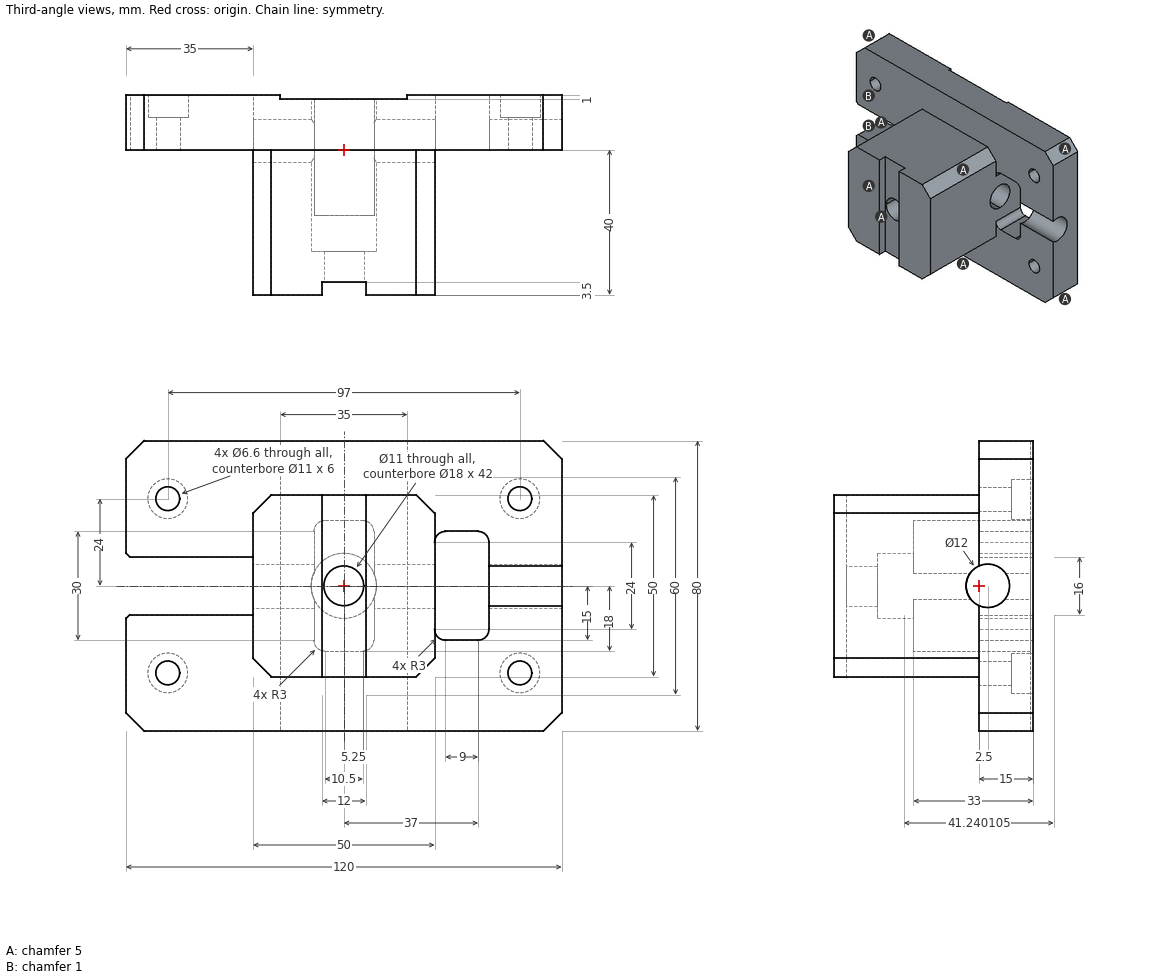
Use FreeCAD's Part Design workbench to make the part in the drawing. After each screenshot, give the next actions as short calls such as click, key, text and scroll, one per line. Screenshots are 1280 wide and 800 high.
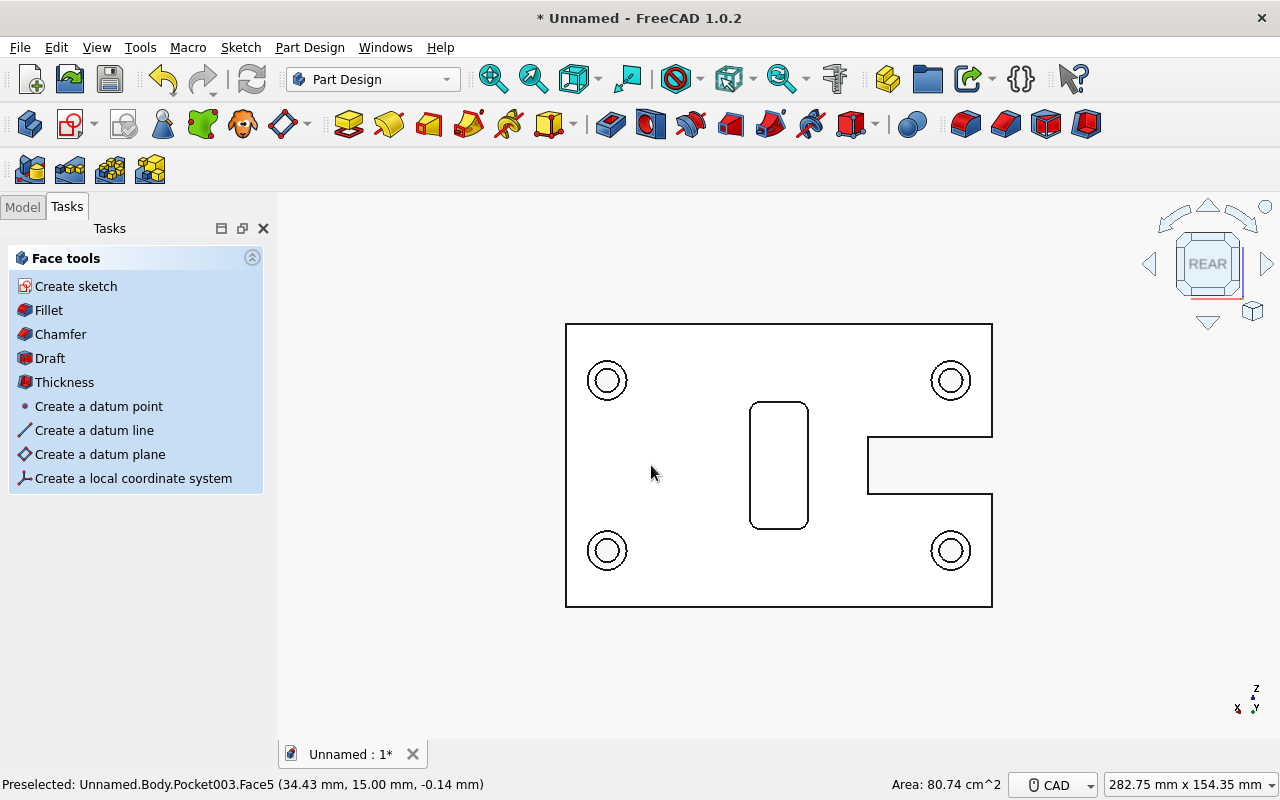
click(70, 124)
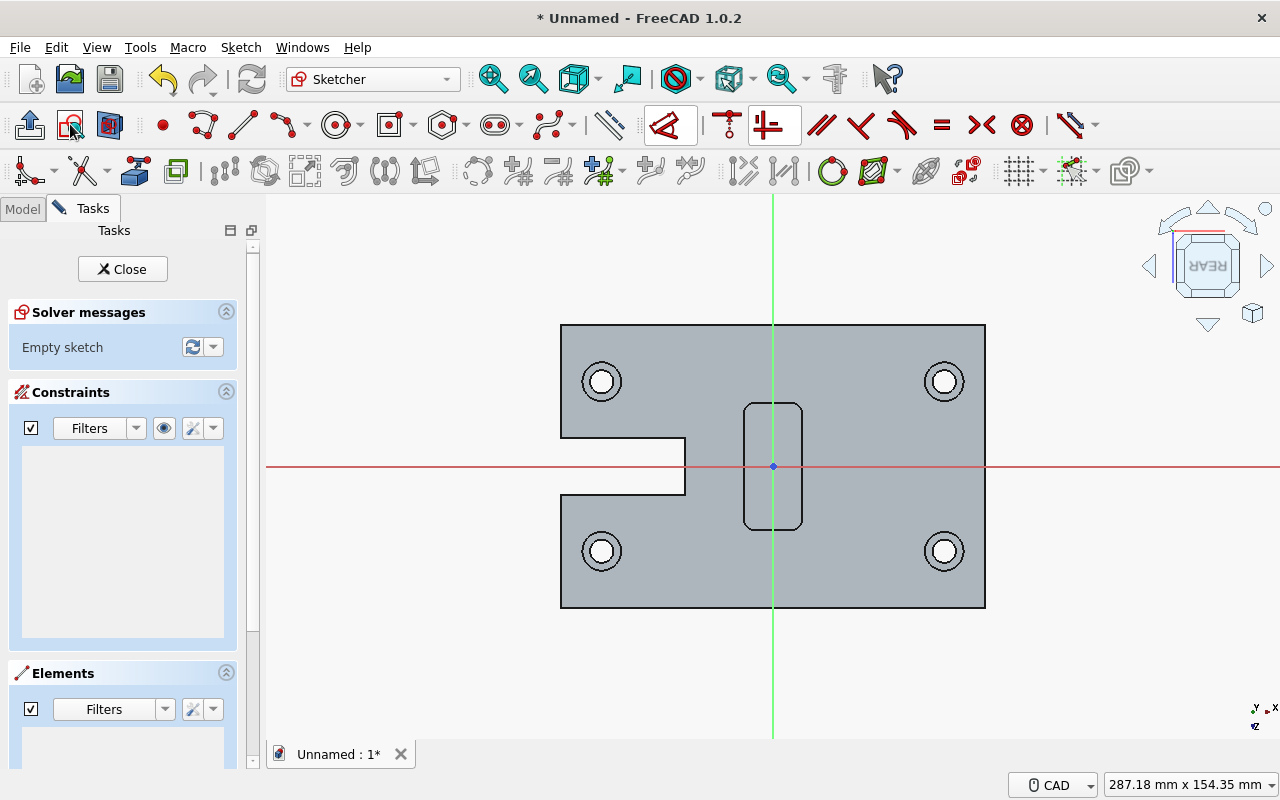
scroll(904, 466, up, 6)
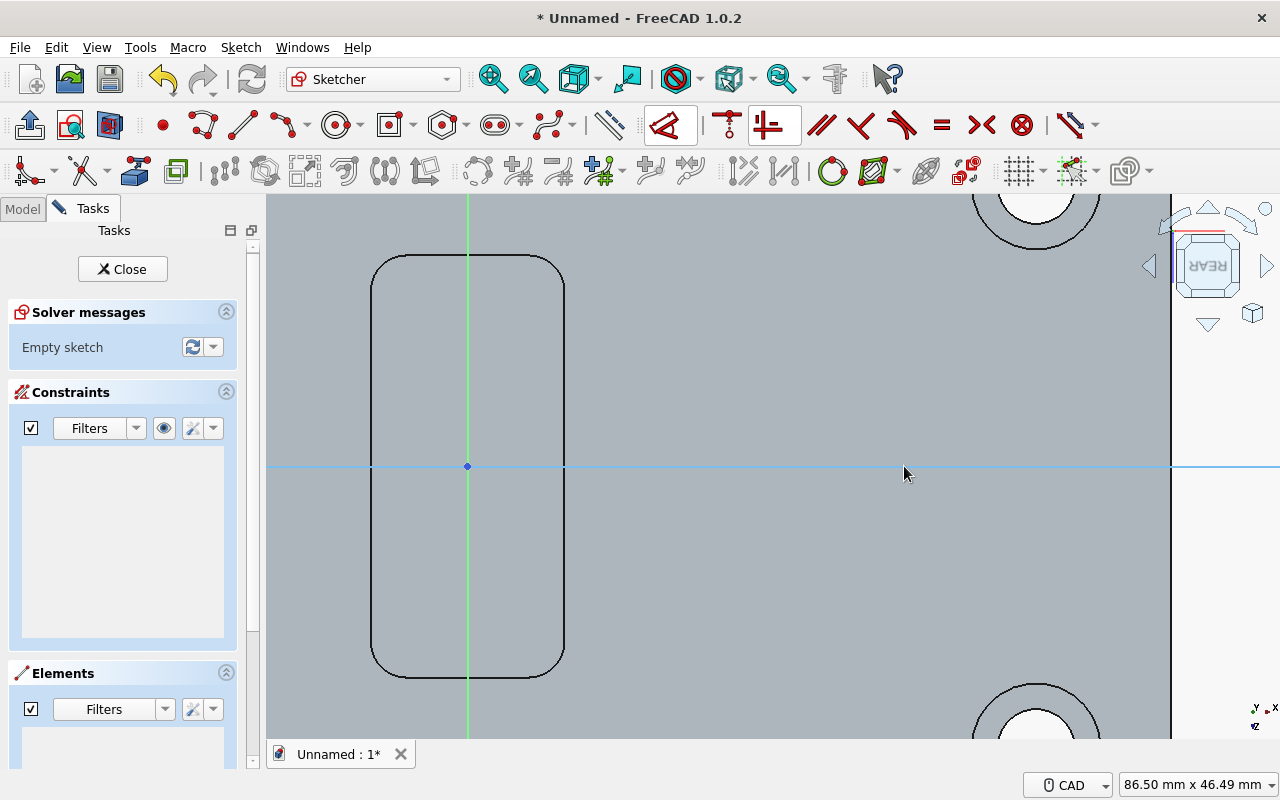
click(244, 126)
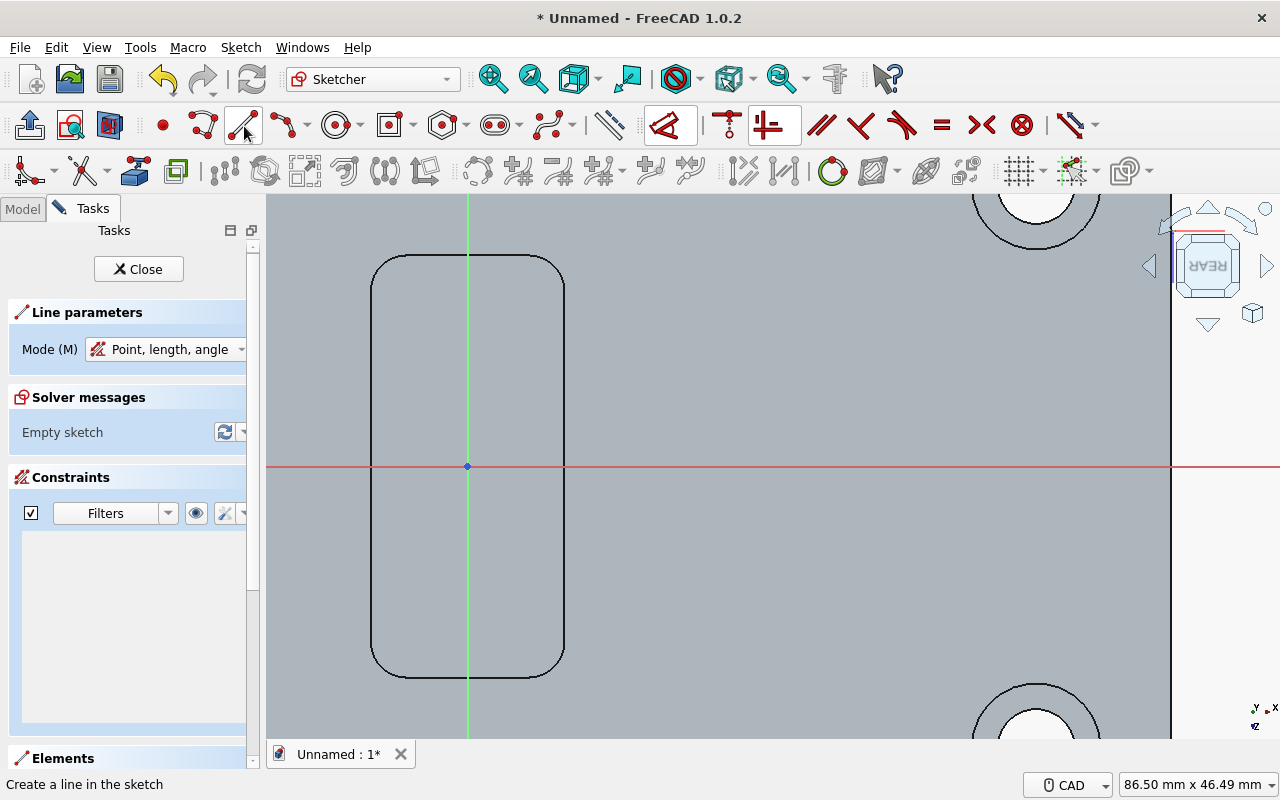
click(901, 291)
click(796, 291)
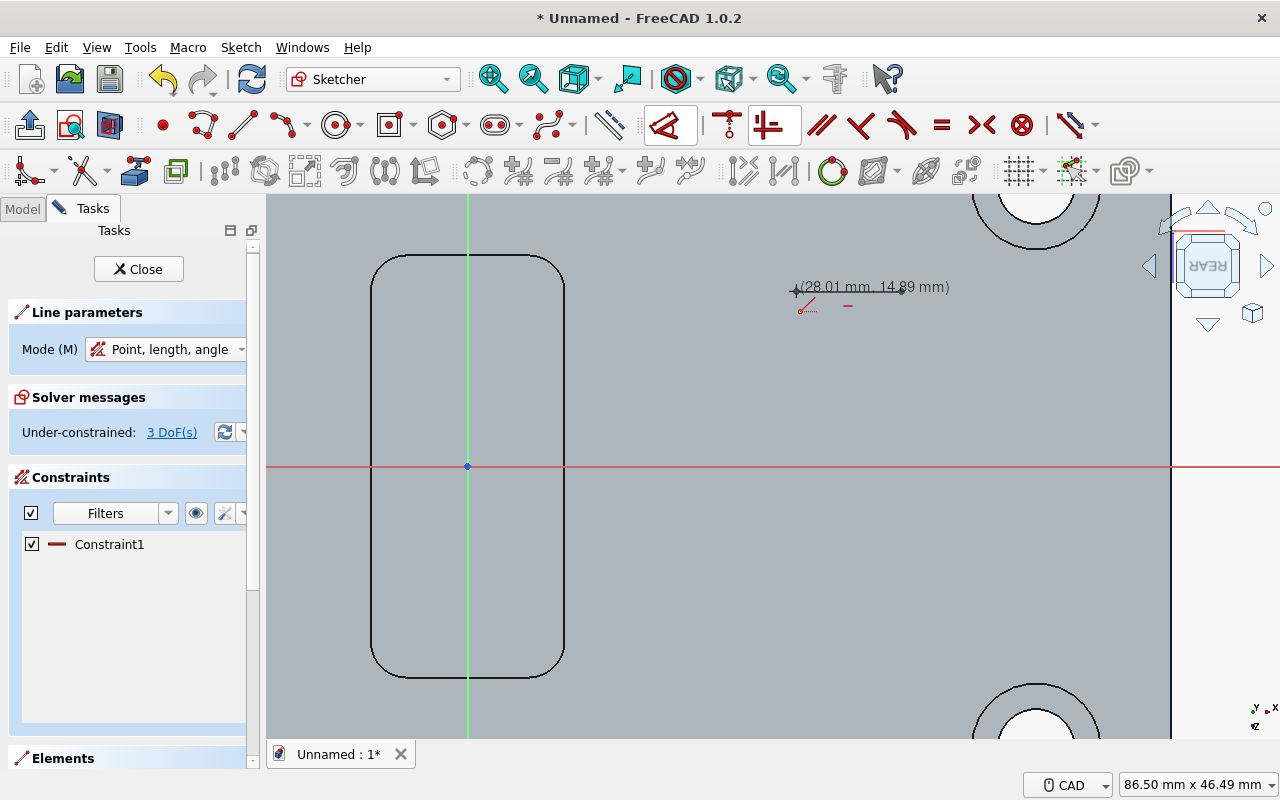
click(761, 326)
click(761, 607)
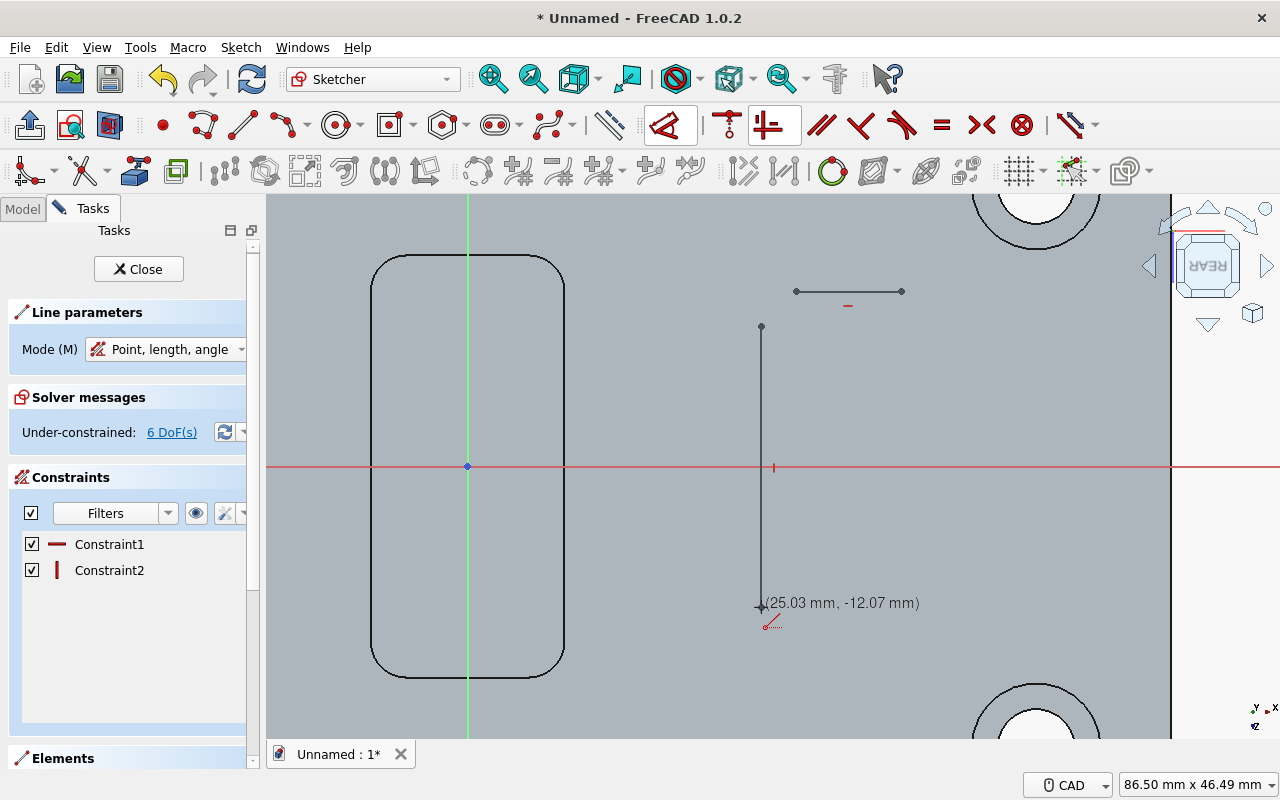
click(796, 642)
click(901, 642)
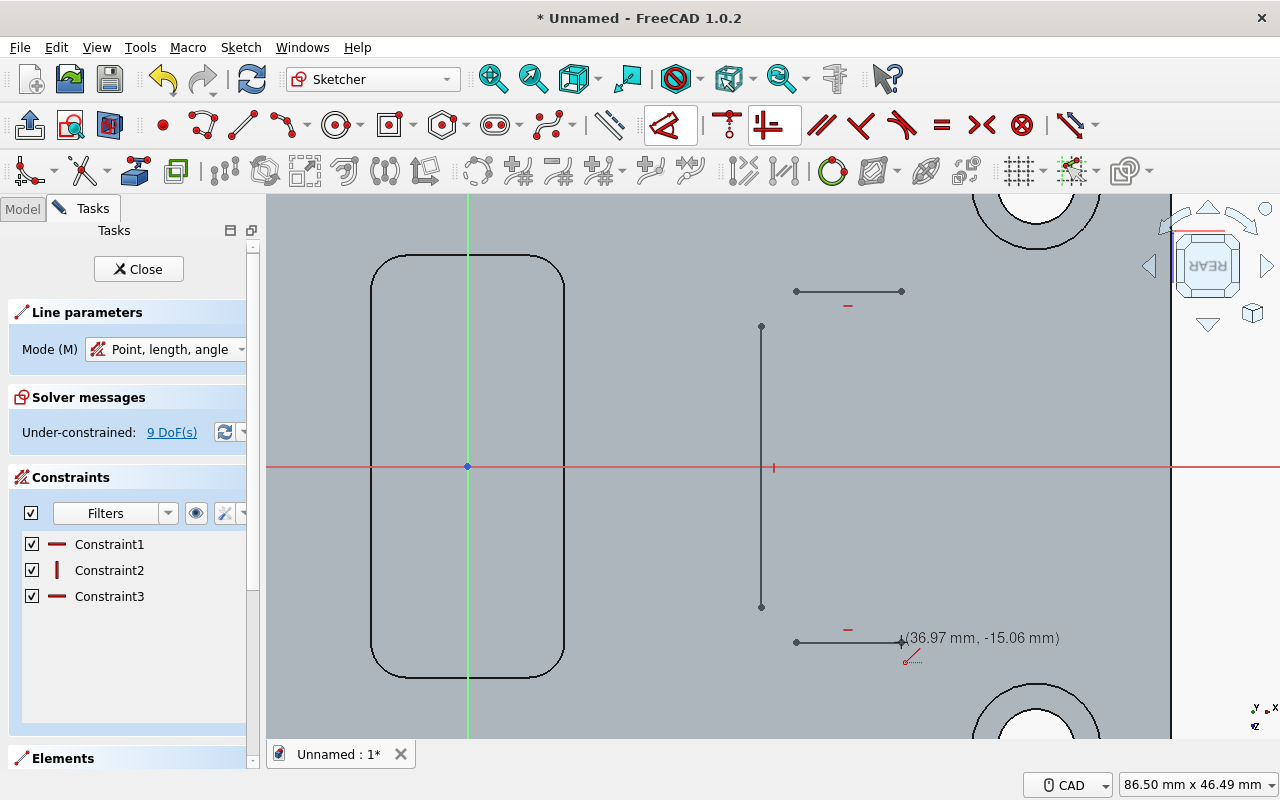
click(937, 607)
click(937, 326)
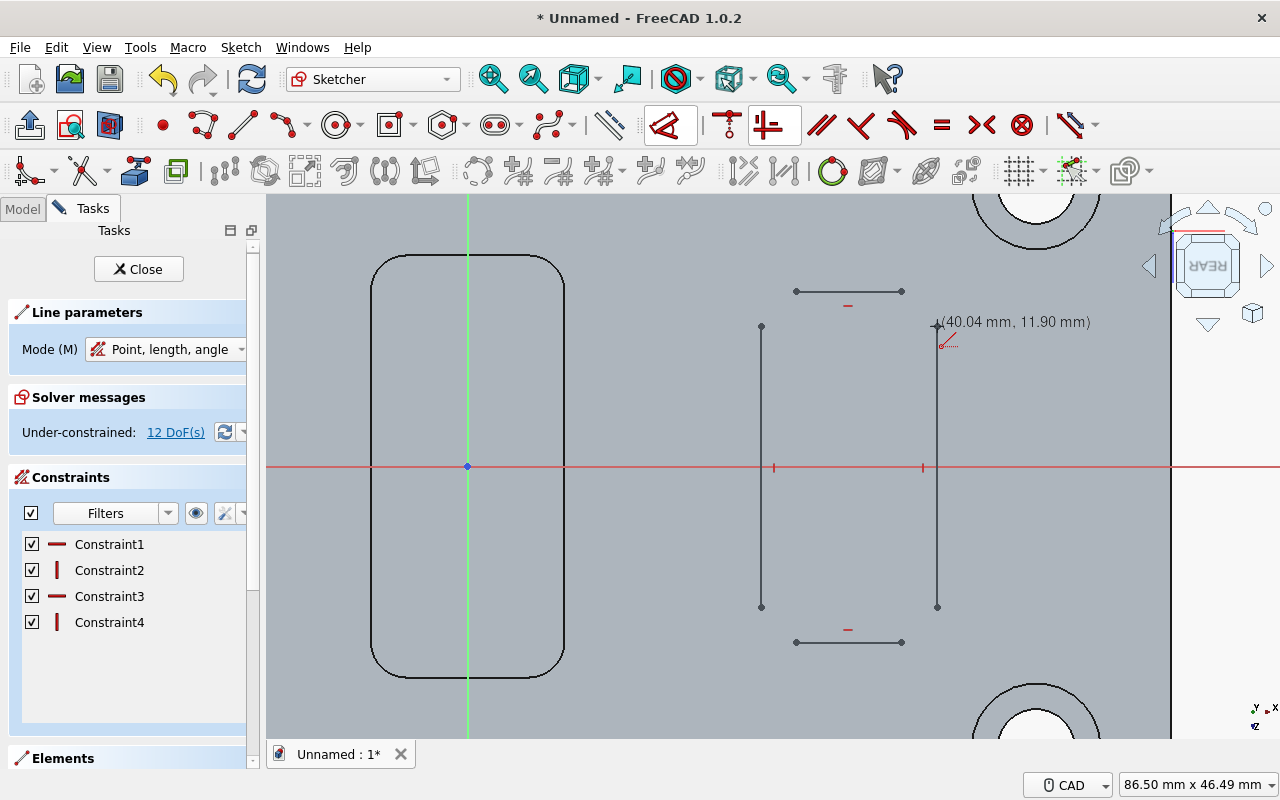
key(g)
key(3)
key(a)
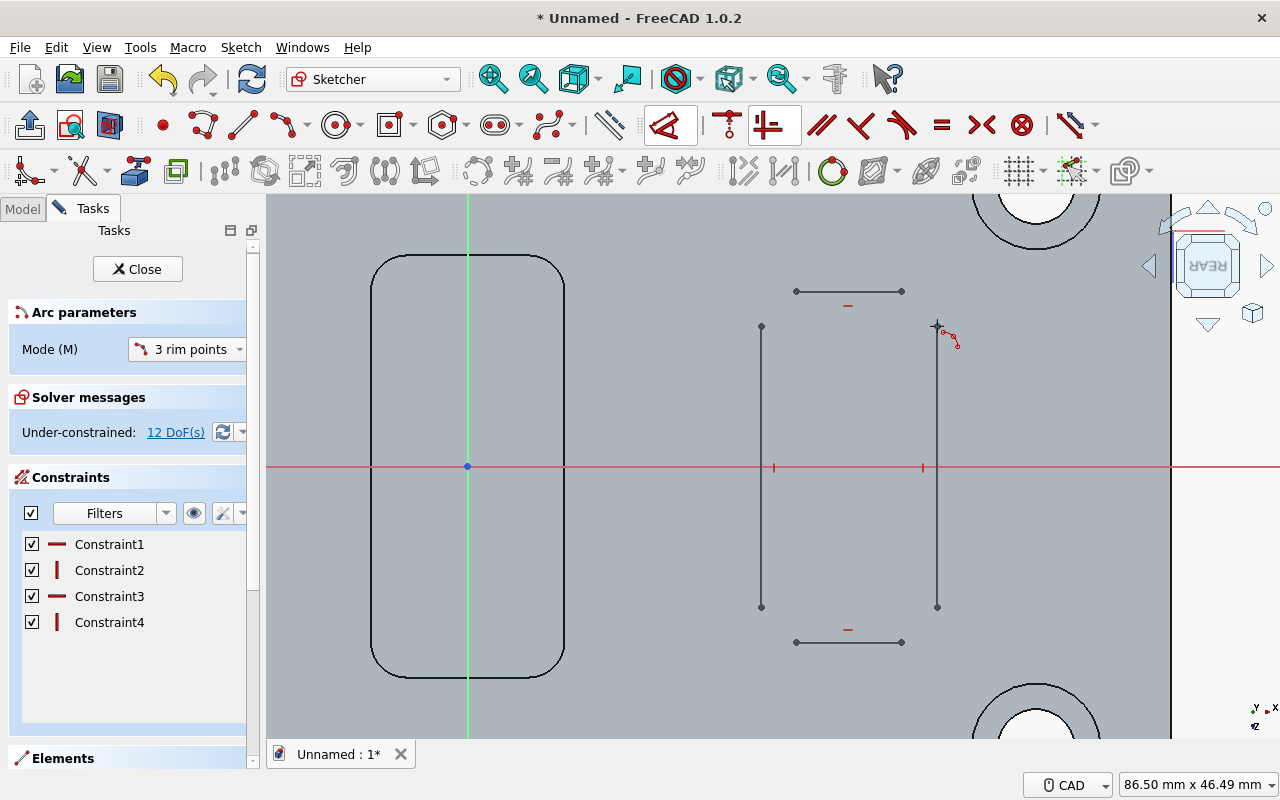
click(796, 292)
click(761, 327)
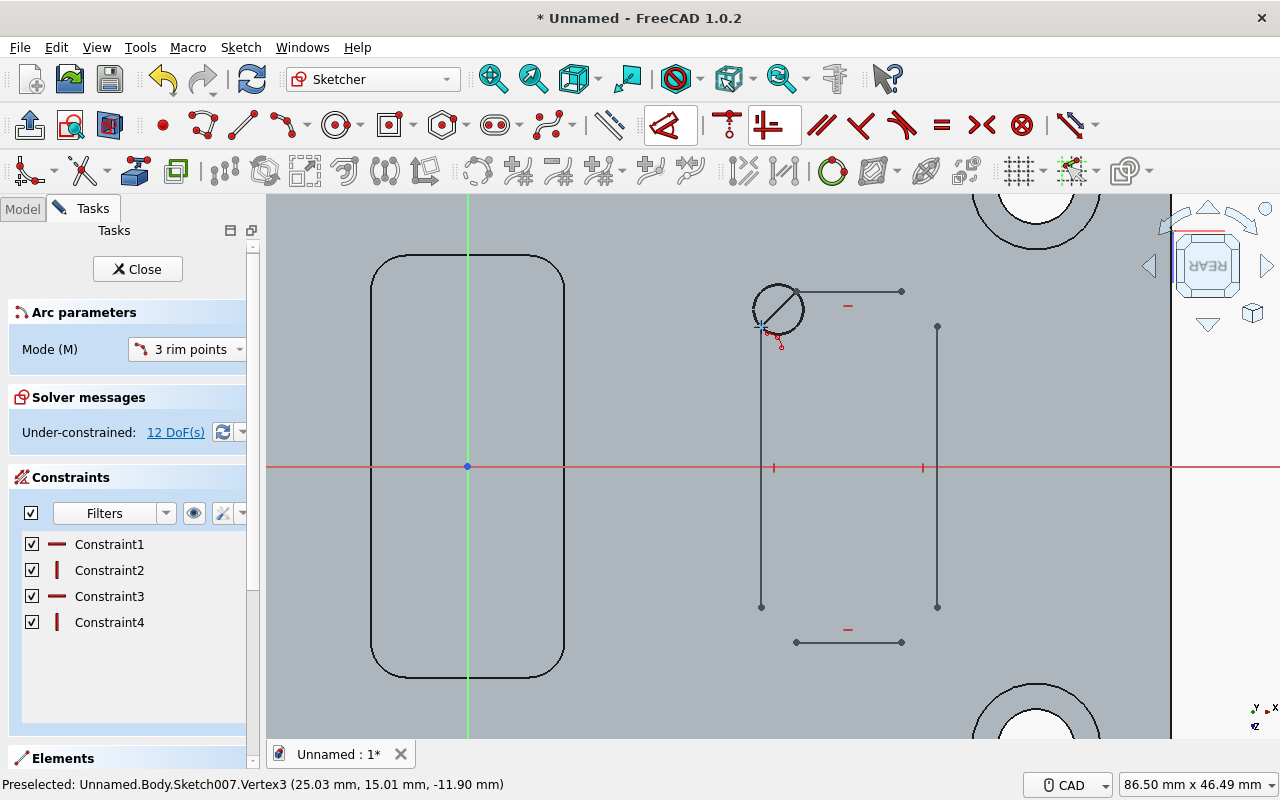
scroll(771, 301, up, 3)